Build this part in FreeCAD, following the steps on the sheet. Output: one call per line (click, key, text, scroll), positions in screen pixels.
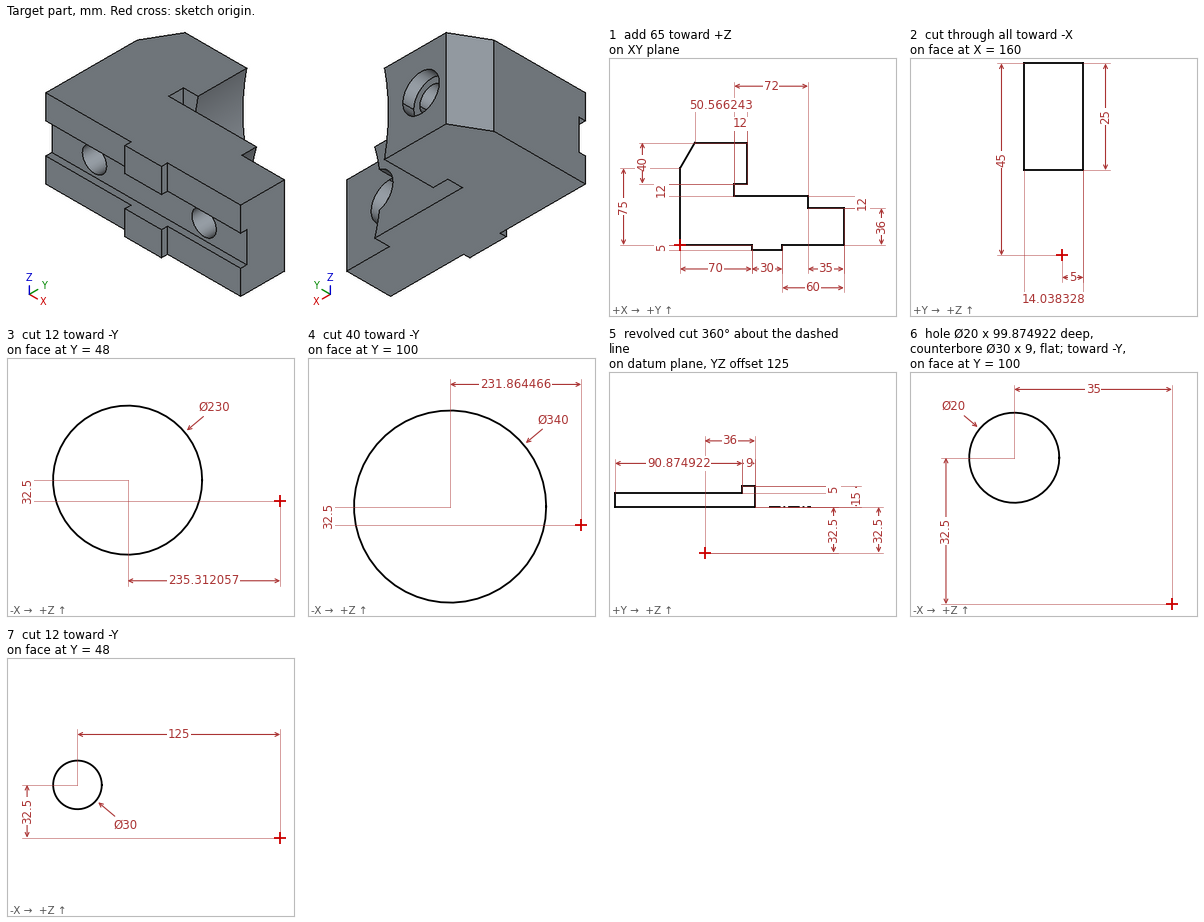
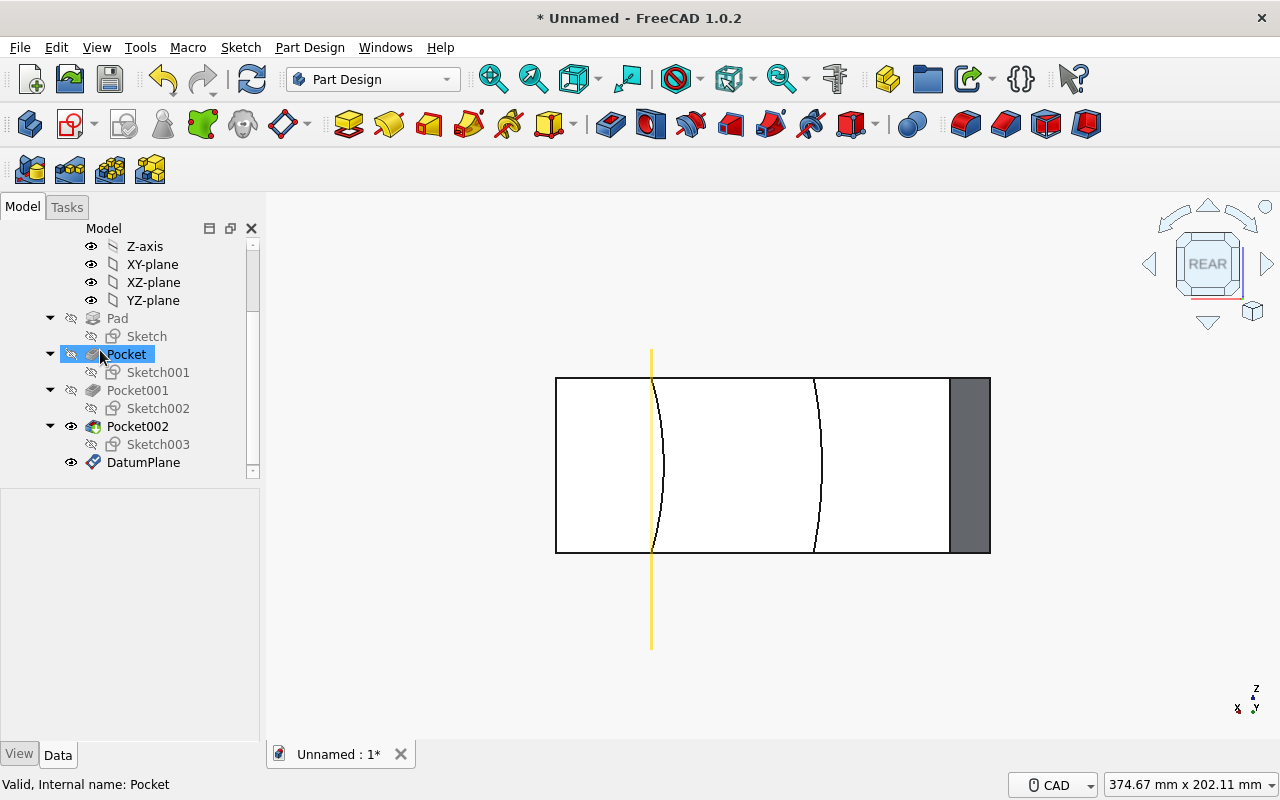
click(116, 462)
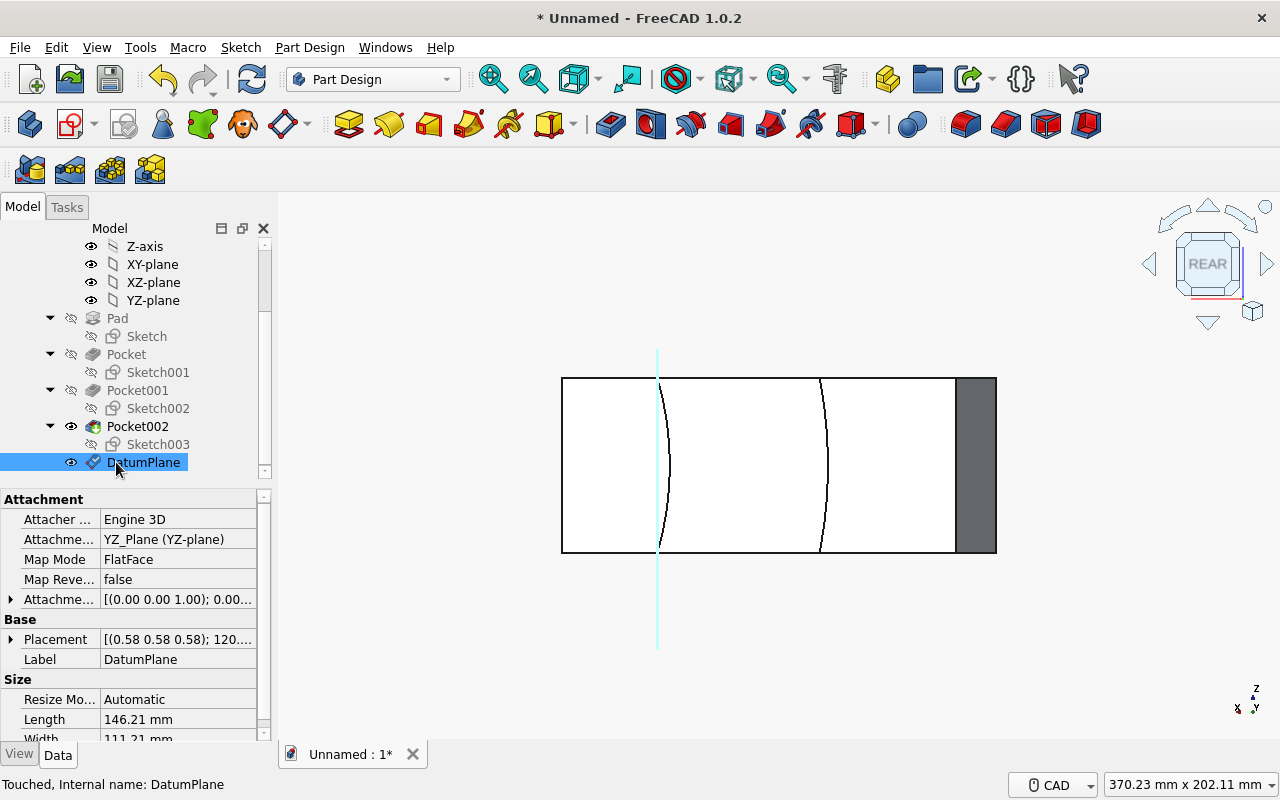
click(70, 124)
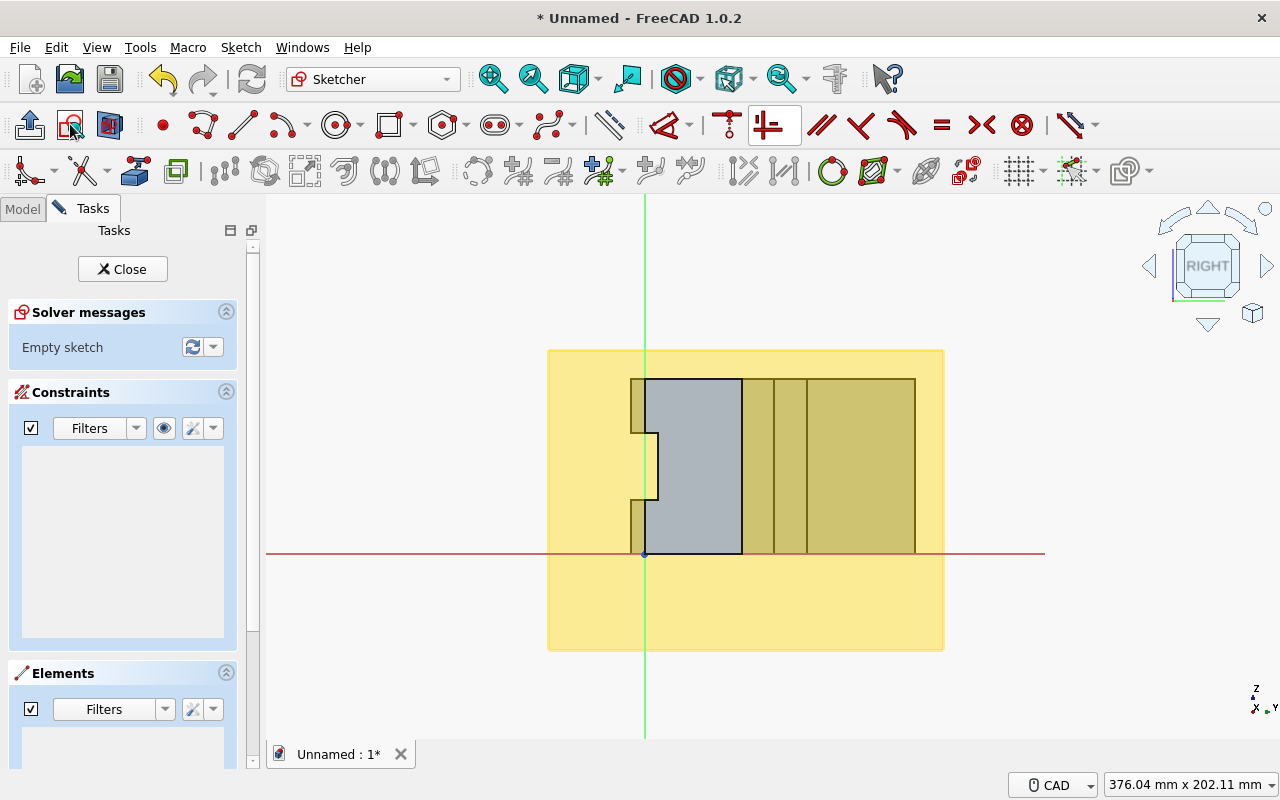
key(q)
key(s)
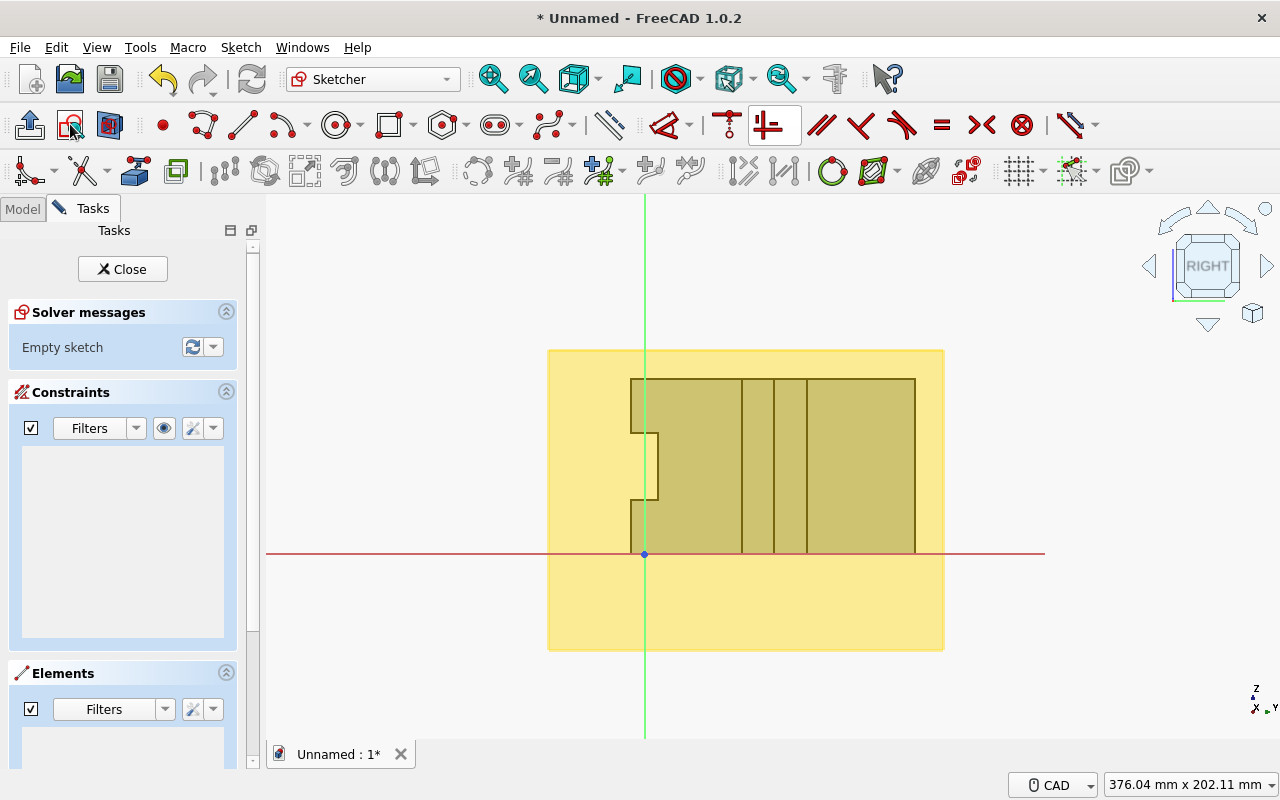
scroll(573, 538, up, 2)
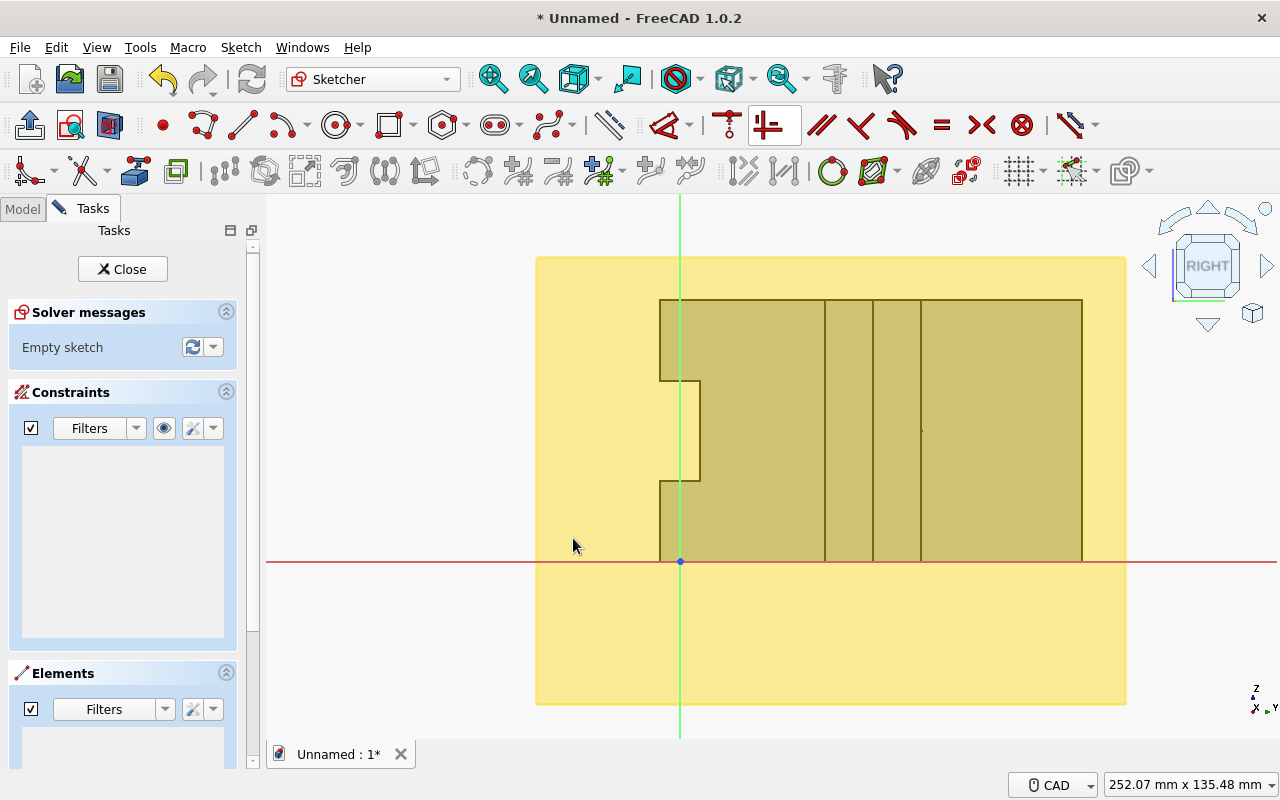
click(204, 126)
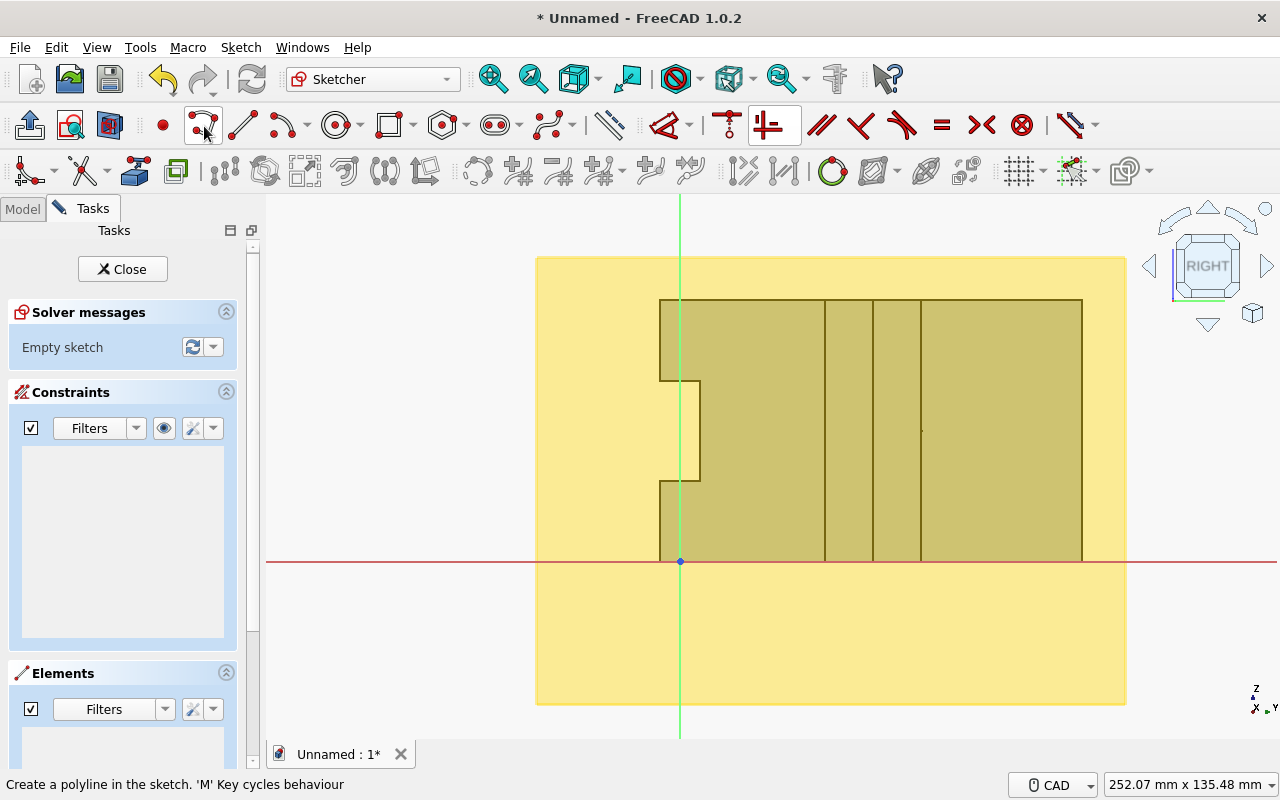
click(825, 431)
click(825, 371)
click(789, 371)
click(789, 391)
click(423, 391)
click(423, 431)
click(825, 432)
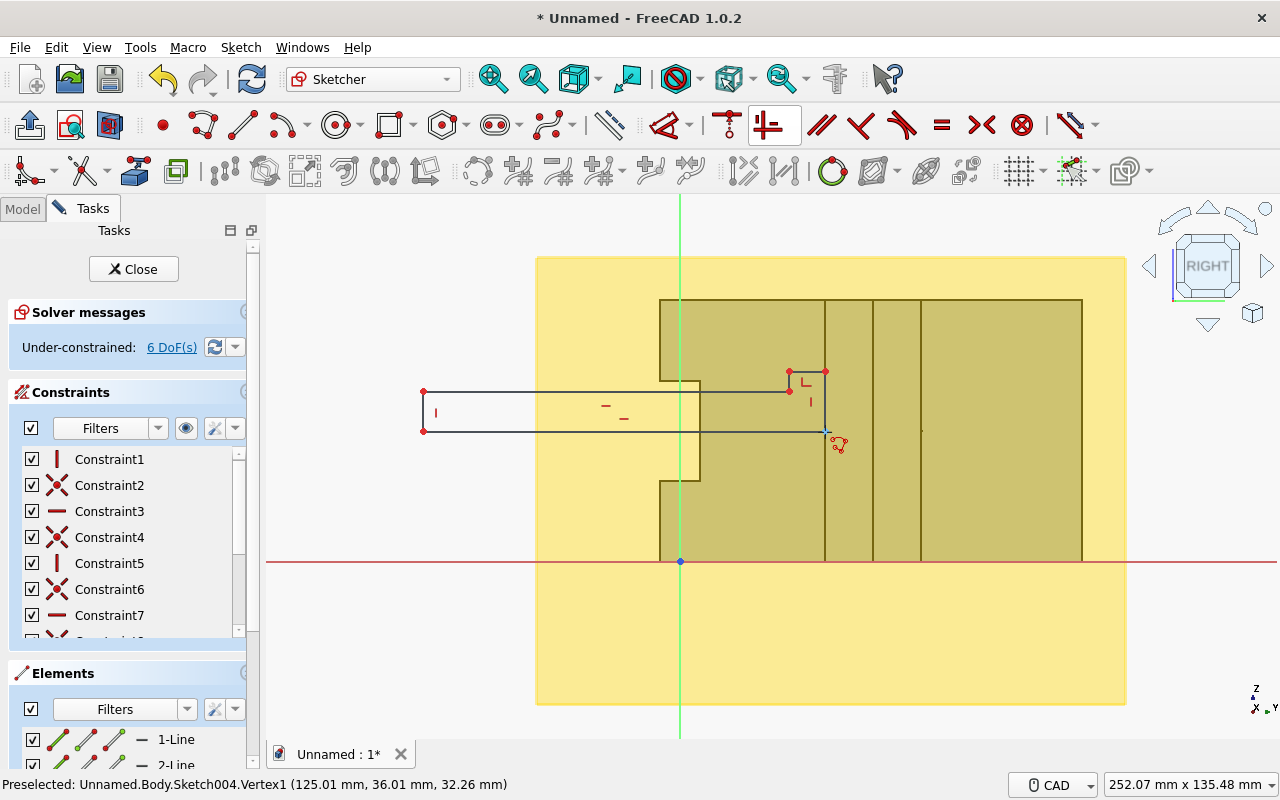
click(244, 126)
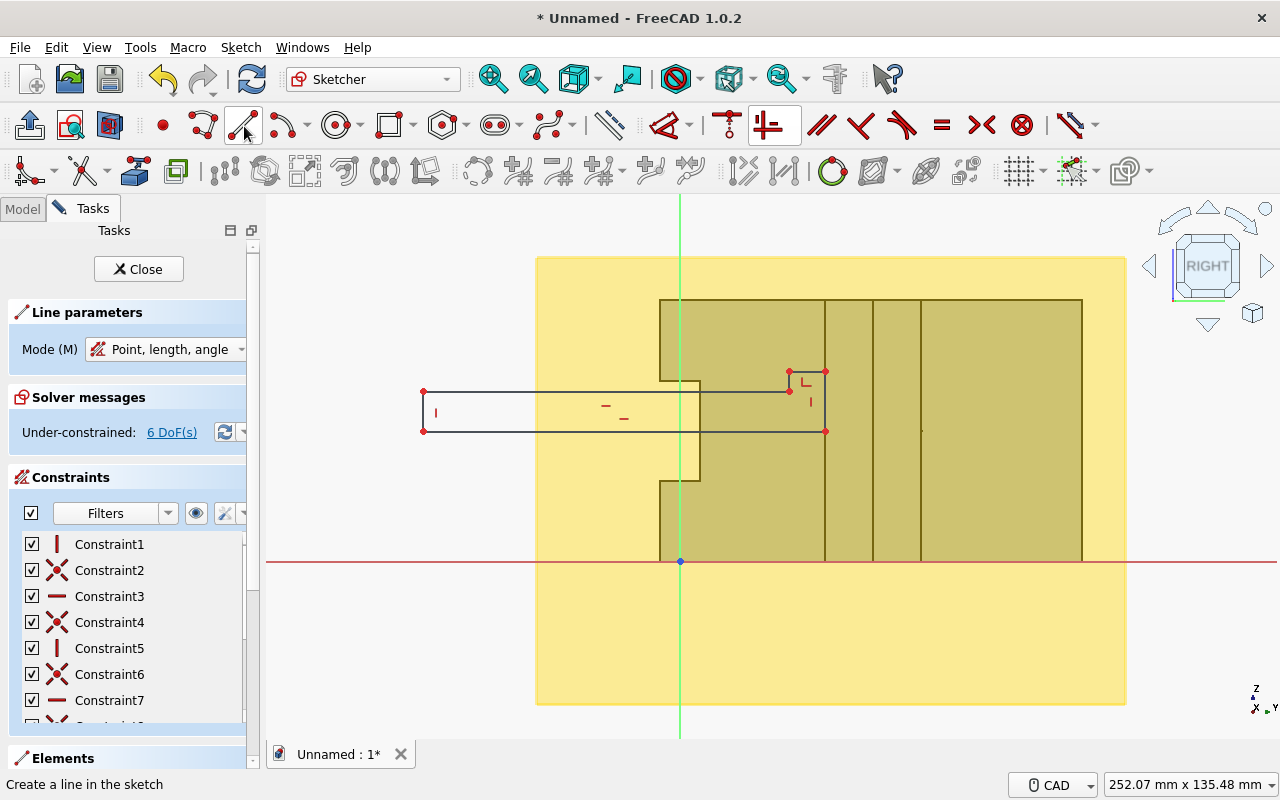
click(865, 431)
click(986, 431)
key(Escape)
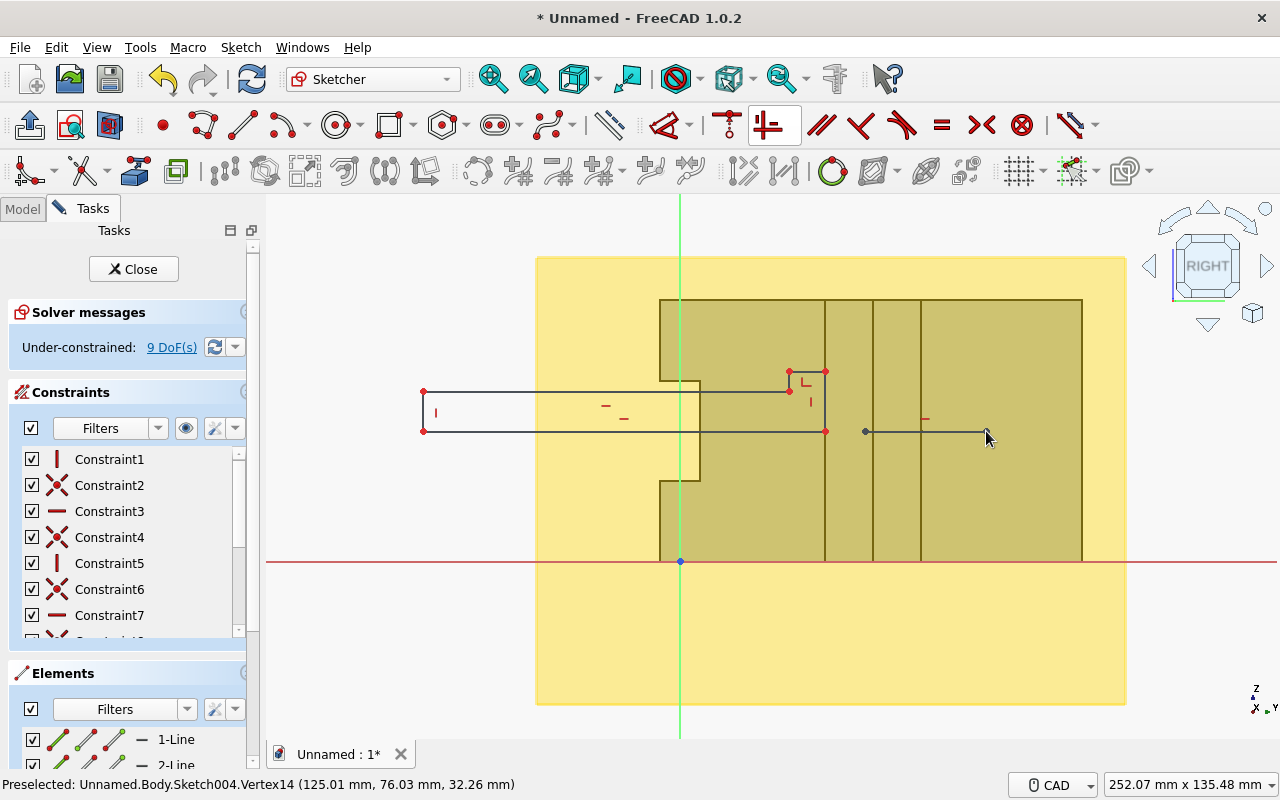
click(901, 432)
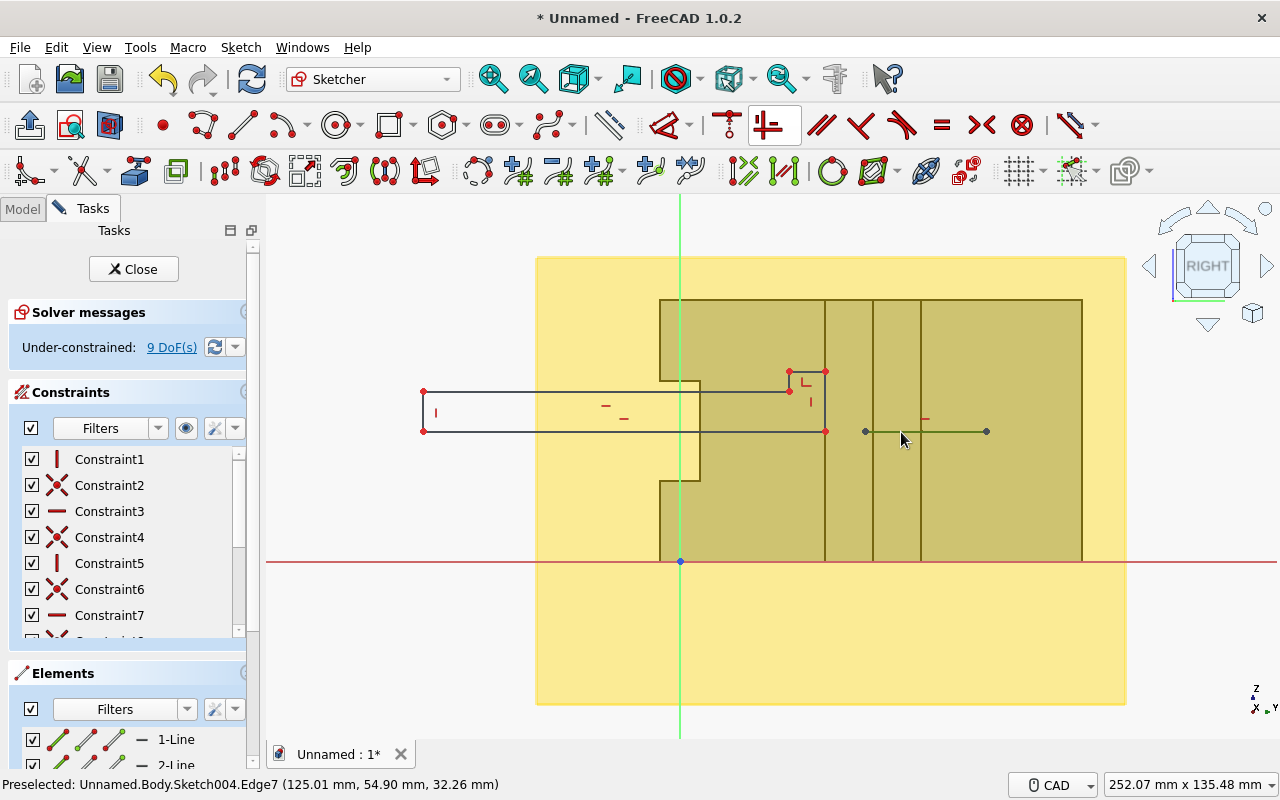
click(610, 126)